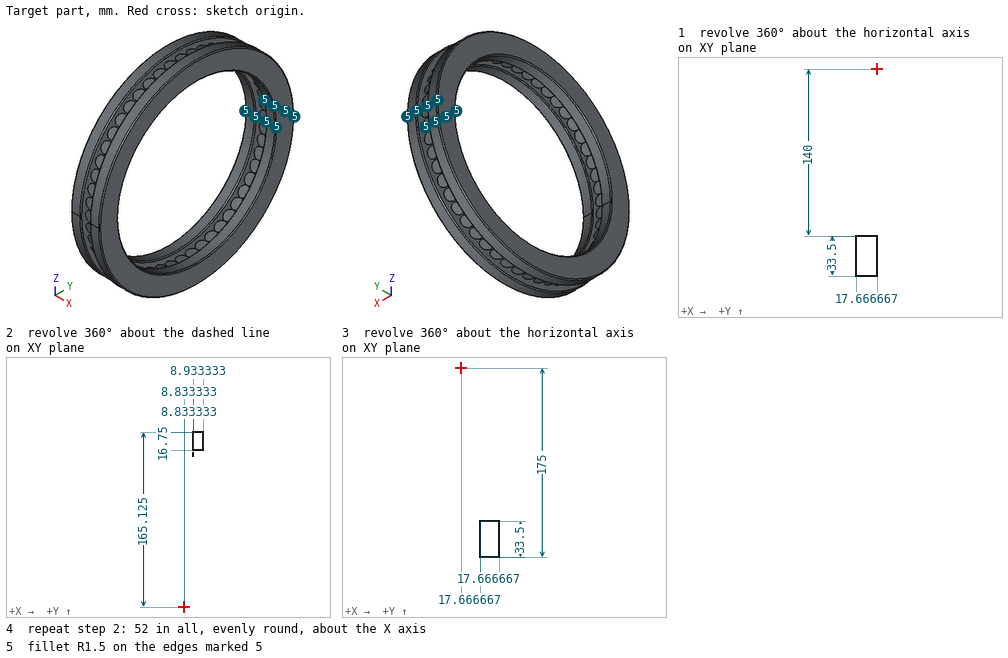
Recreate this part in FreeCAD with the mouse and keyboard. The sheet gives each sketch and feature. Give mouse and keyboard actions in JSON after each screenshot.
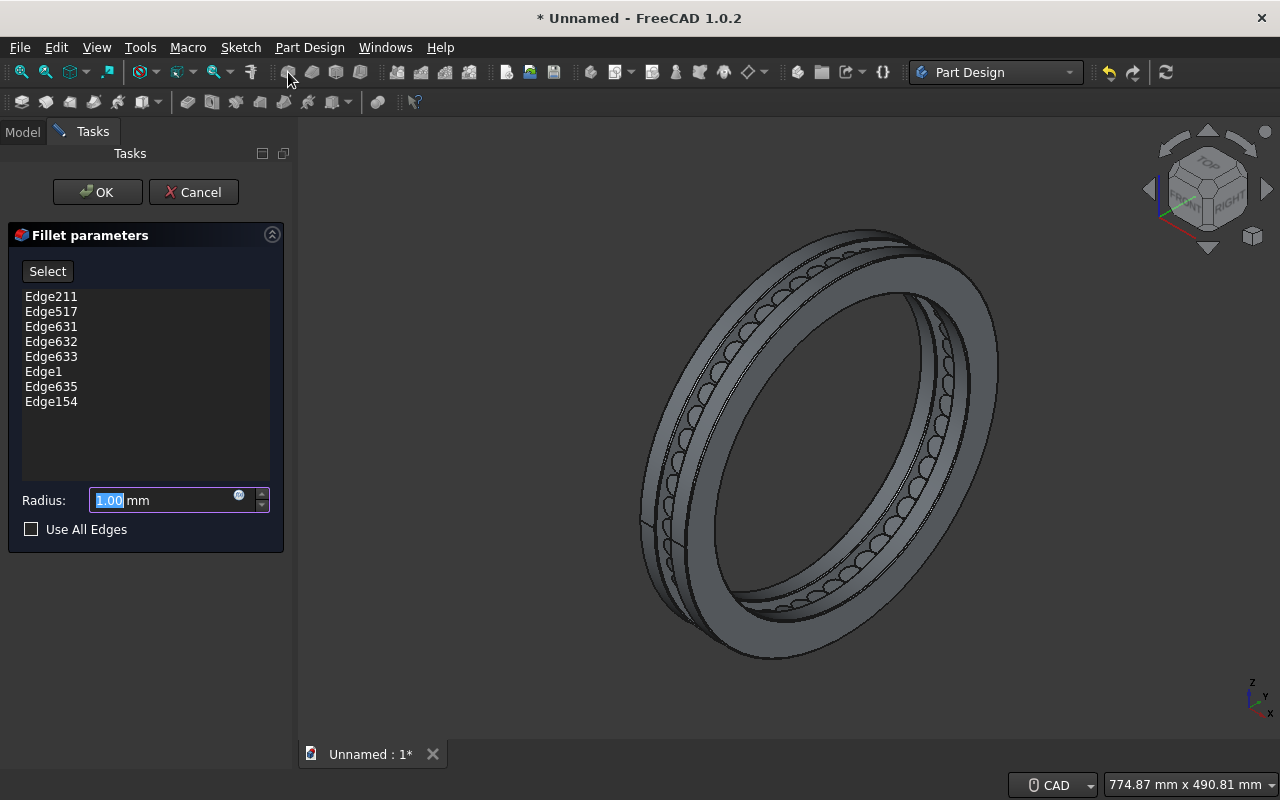
{"action": "type", "text": "1.5"}
{"action": "key", "text": "Tab"}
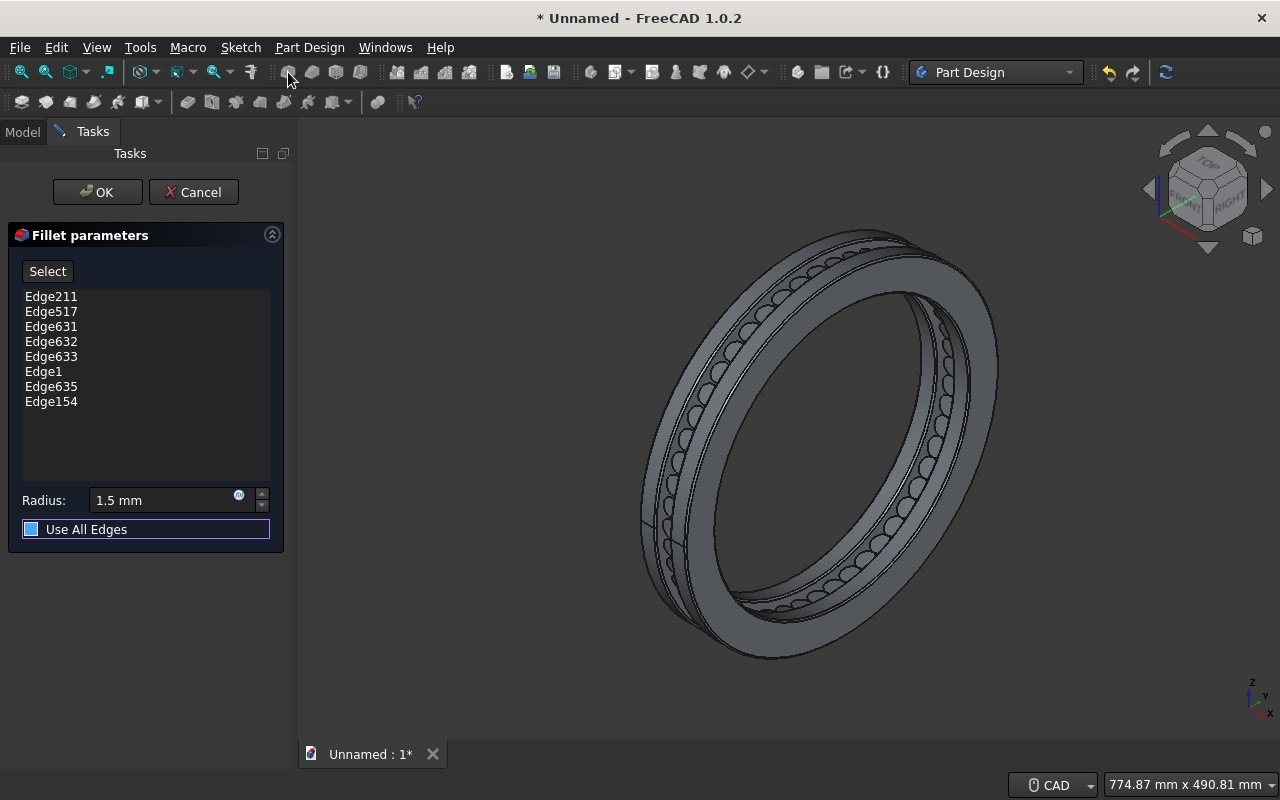
{"action": "left_click", "coordinate": [98, 192]}